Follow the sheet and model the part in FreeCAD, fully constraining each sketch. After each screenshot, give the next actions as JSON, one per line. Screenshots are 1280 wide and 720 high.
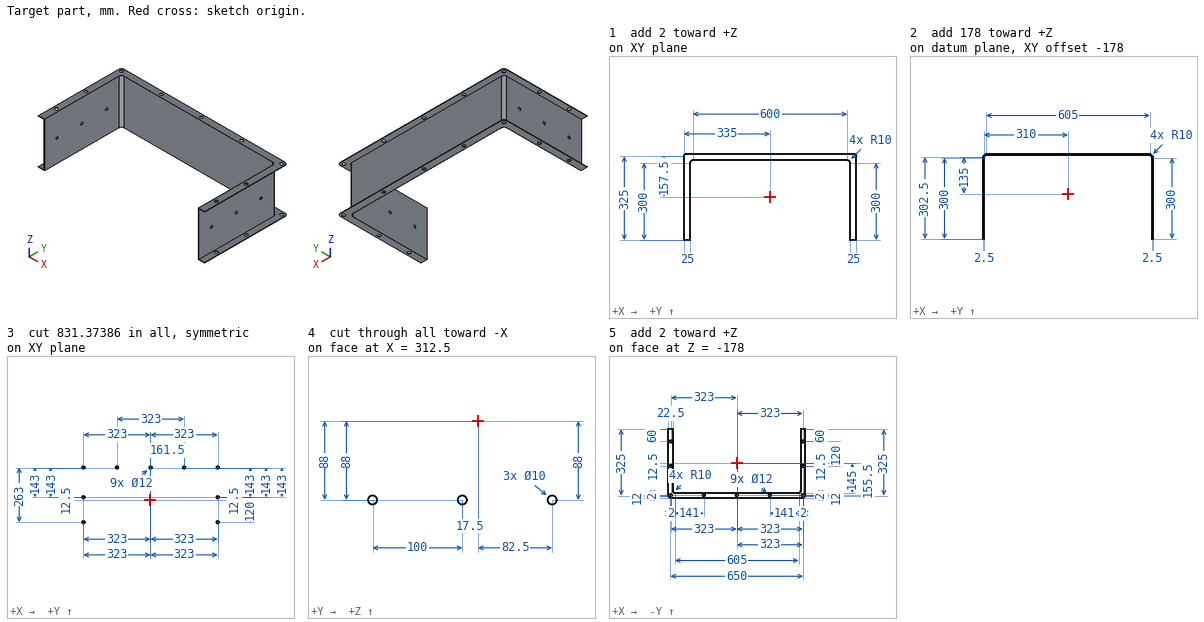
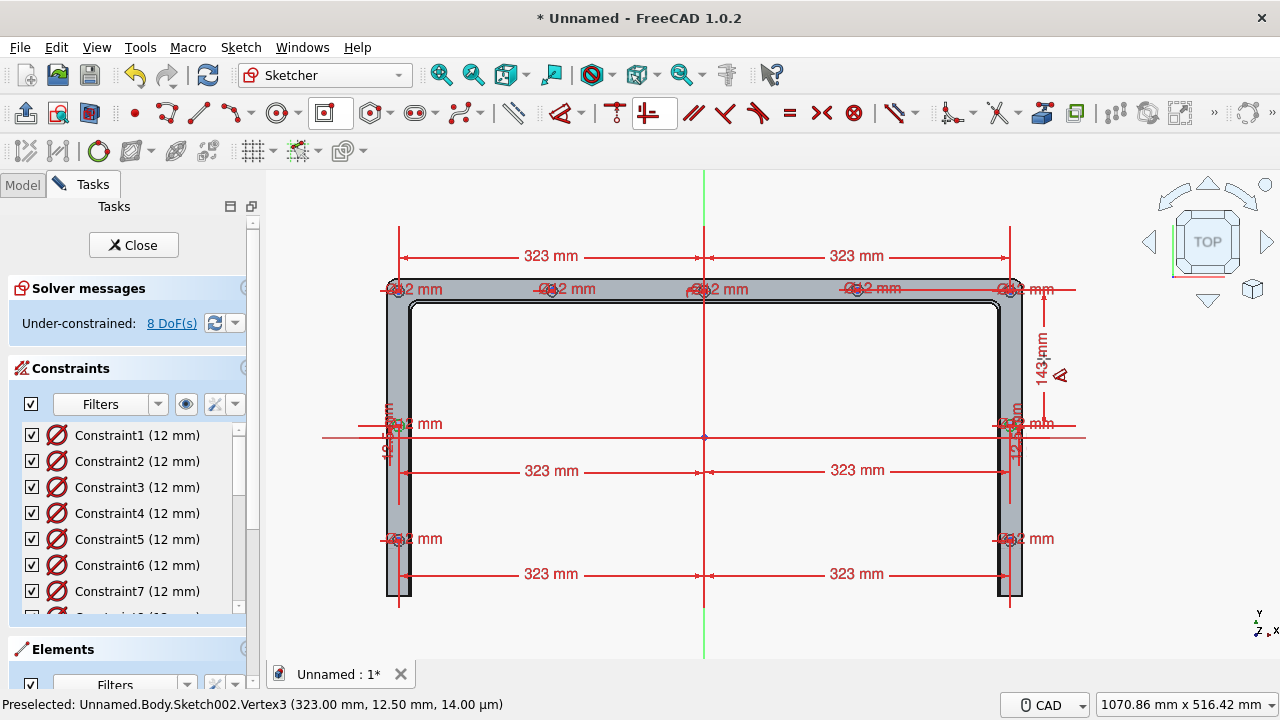
{"action": "left_click", "coordinate": [704, 291]}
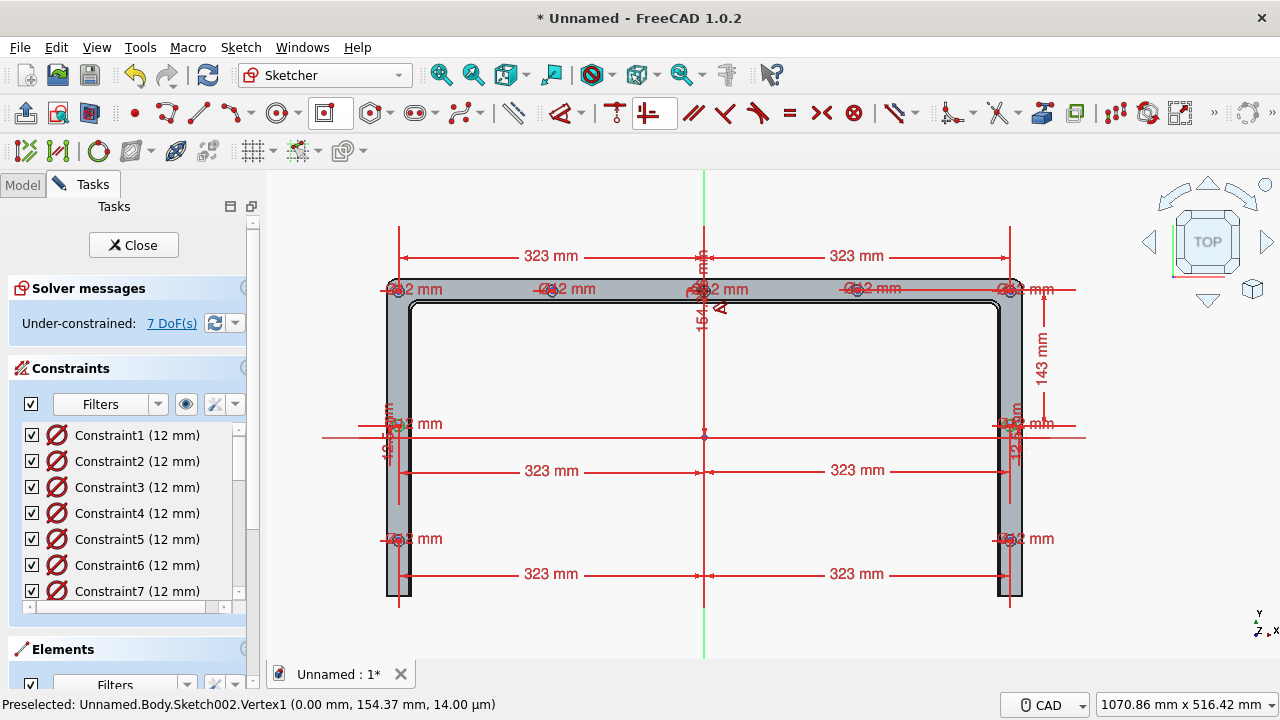
{"action": "left_click", "coordinate": [1010, 426]}
{"action": "left_click", "coordinate": [1044, 328]}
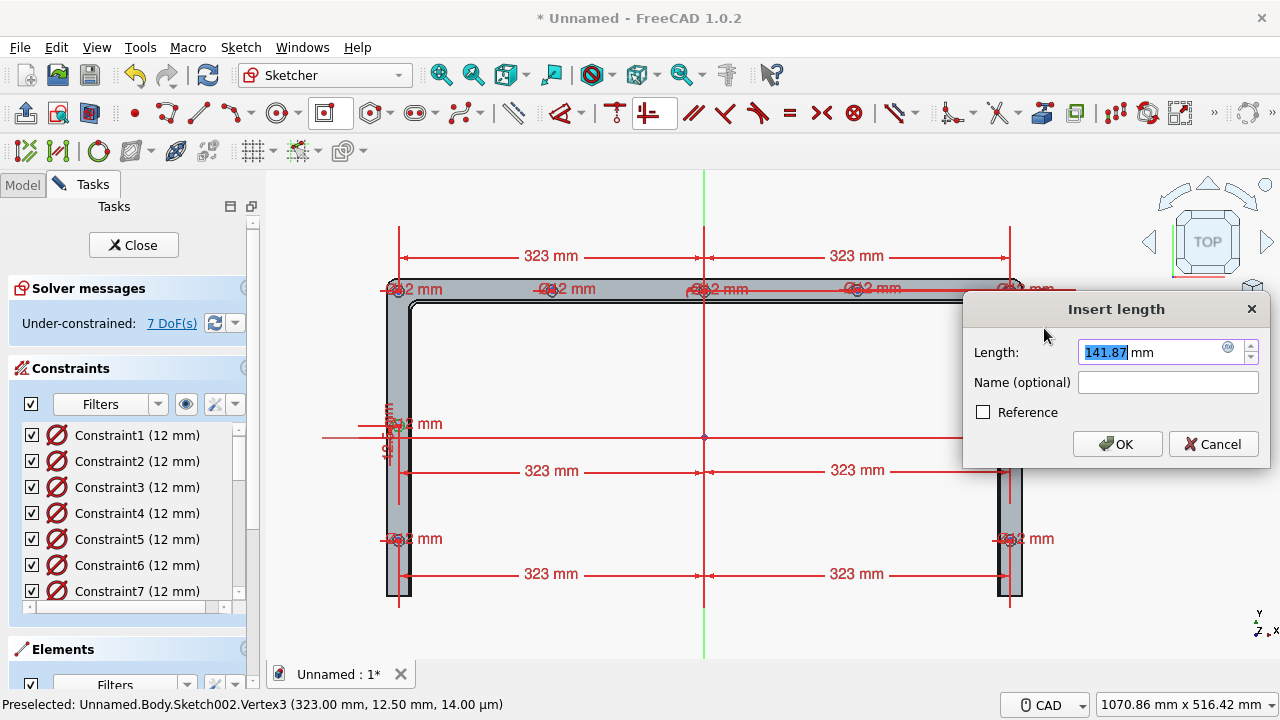
{"action": "type", "text": "143"}
{"action": "key", "text": "Return"}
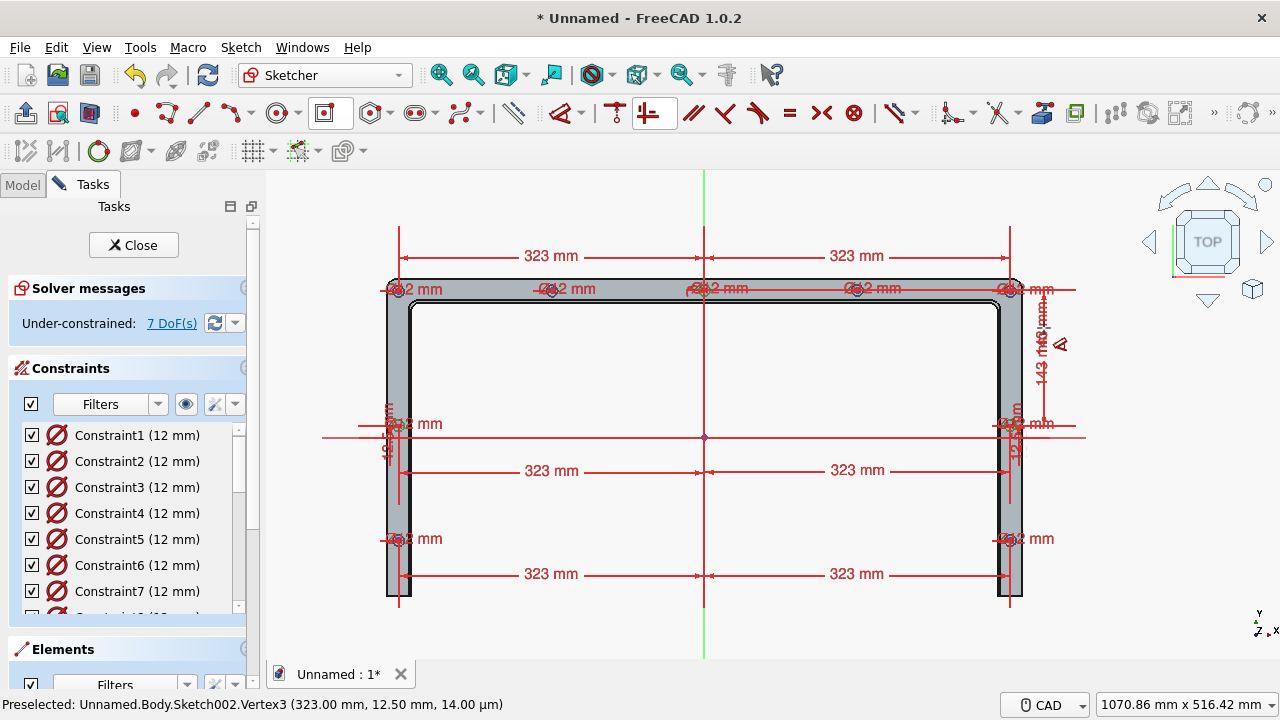
{"action": "left_click", "coordinate": [1010, 426]}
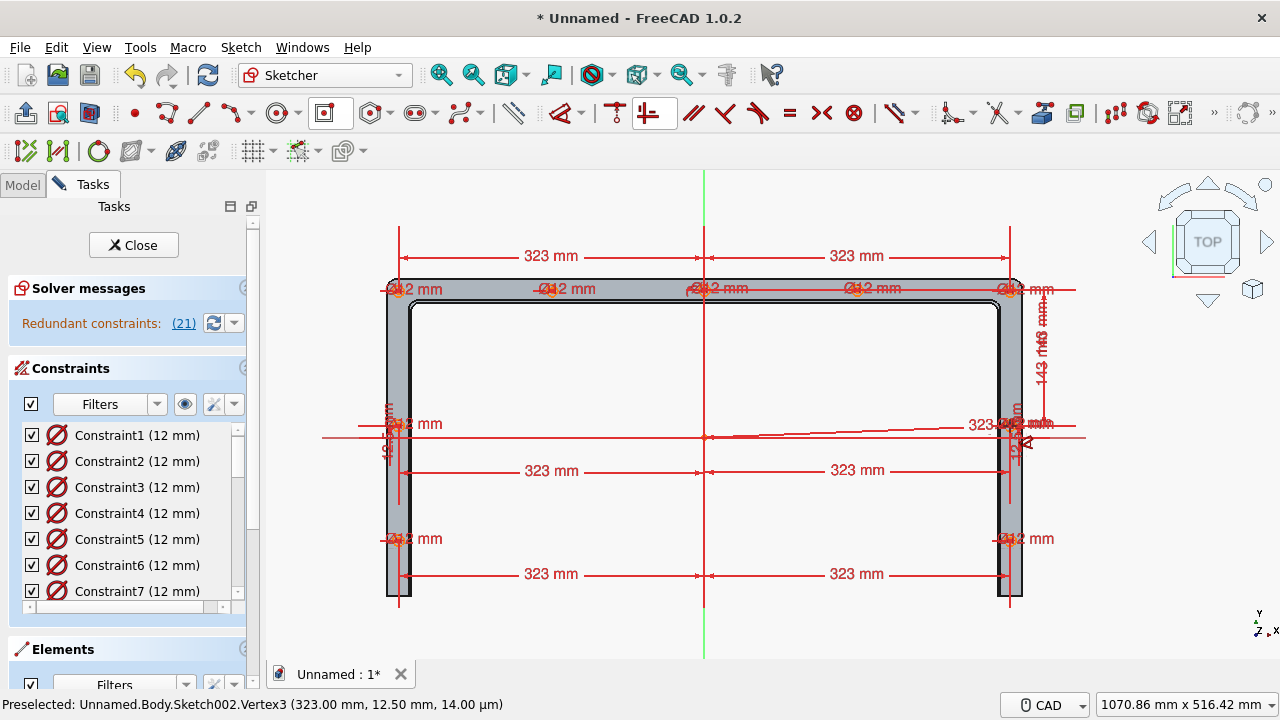
{"action": "left_click", "coordinate": [1010, 541]}
{"action": "left_click", "coordinate": [1044, 483]}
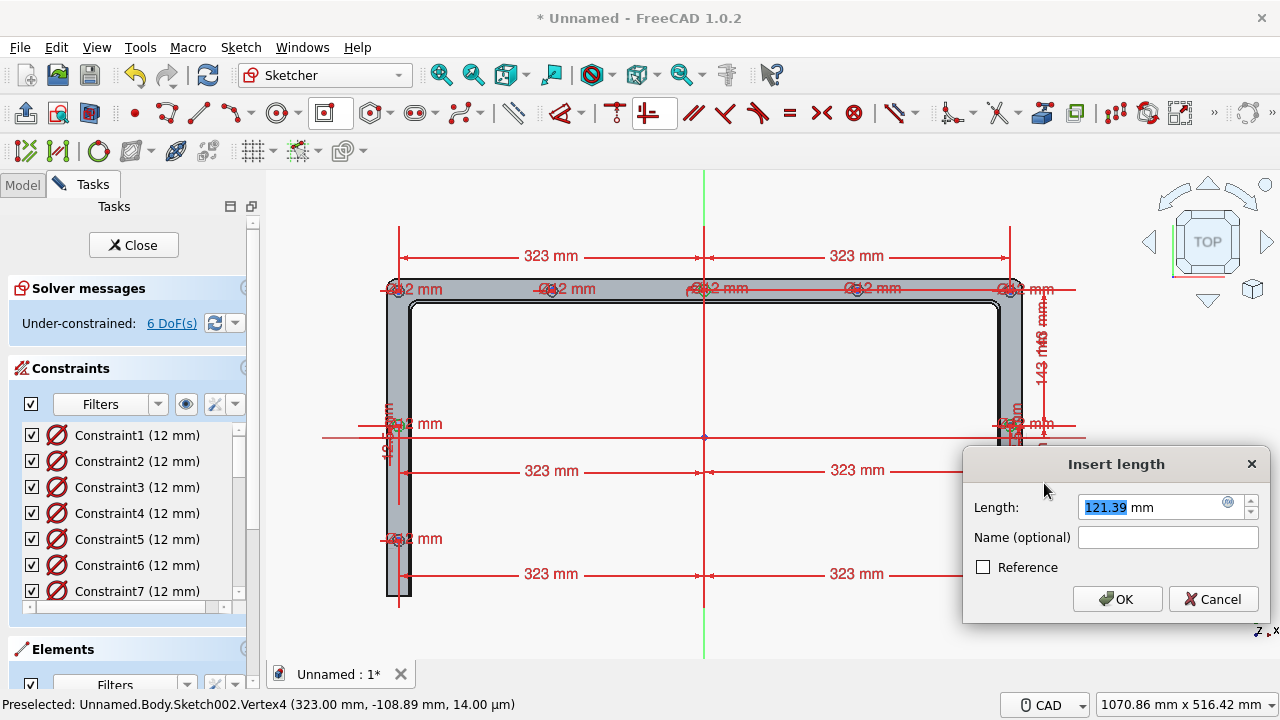
{"action": "type", "text": "120"}
{"action": "key", "text": "Return"}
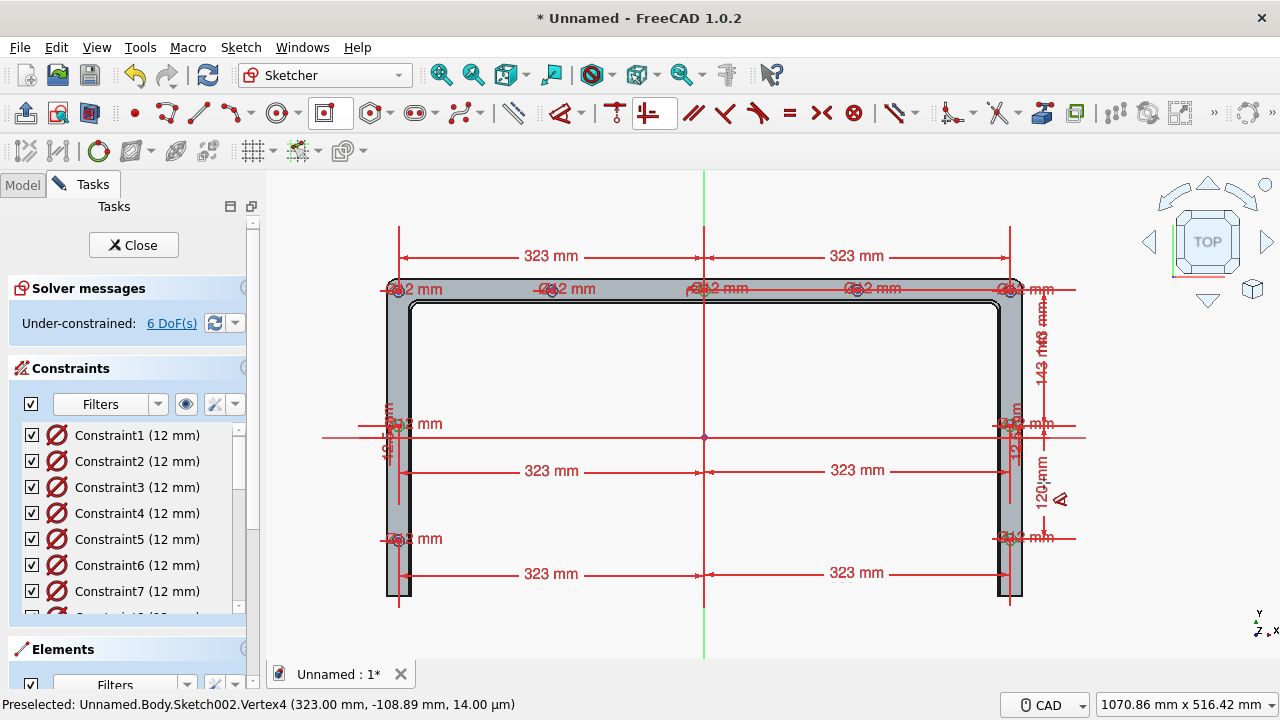
{"action": "left_click", "coordinate": [1010, 426]}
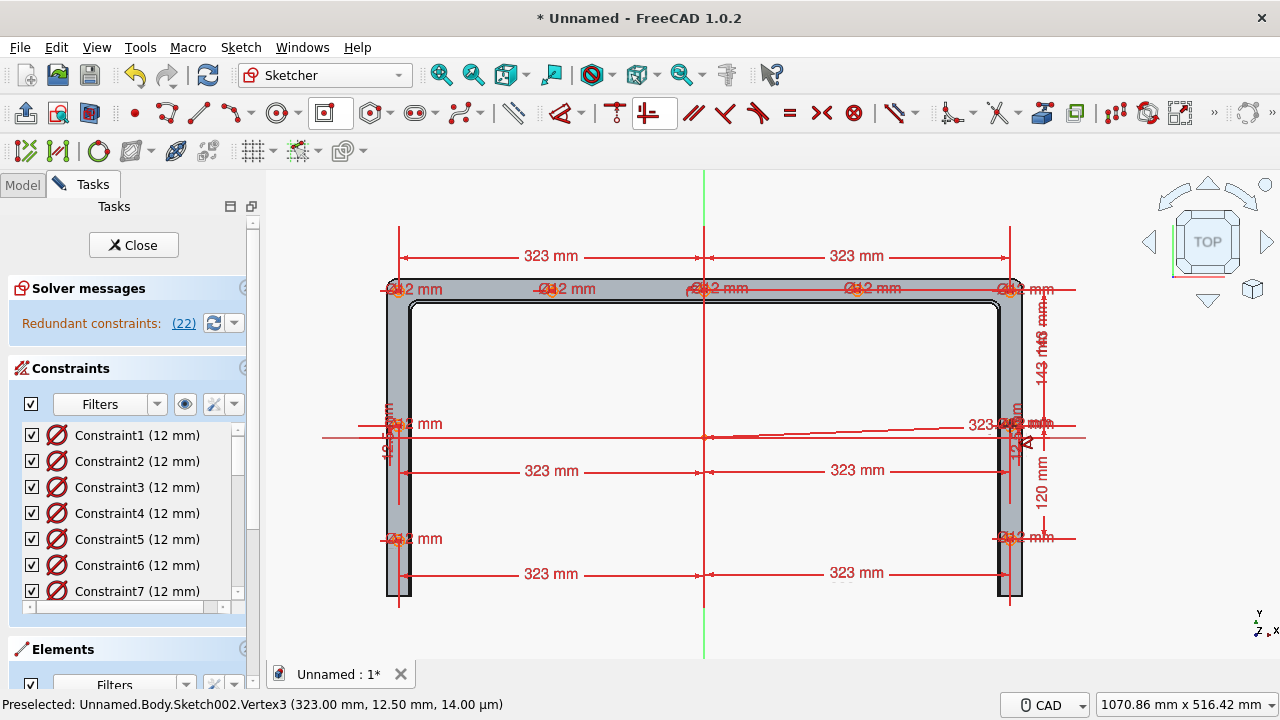
{"action": "left_click", "coordinate": [1010, 291]}
{"action": "left_click", "coordinate": [1044, 389]}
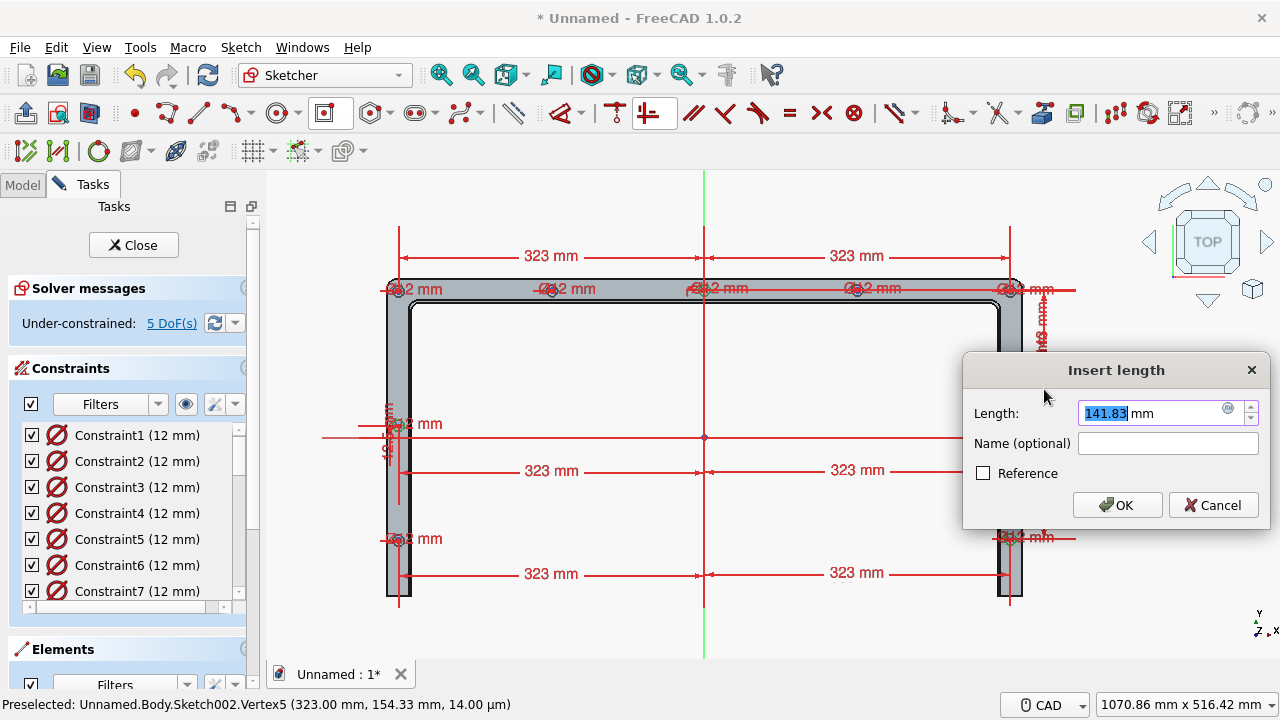
{"action": "type", "text": "143"}
{"action": "key", "text": "Return"}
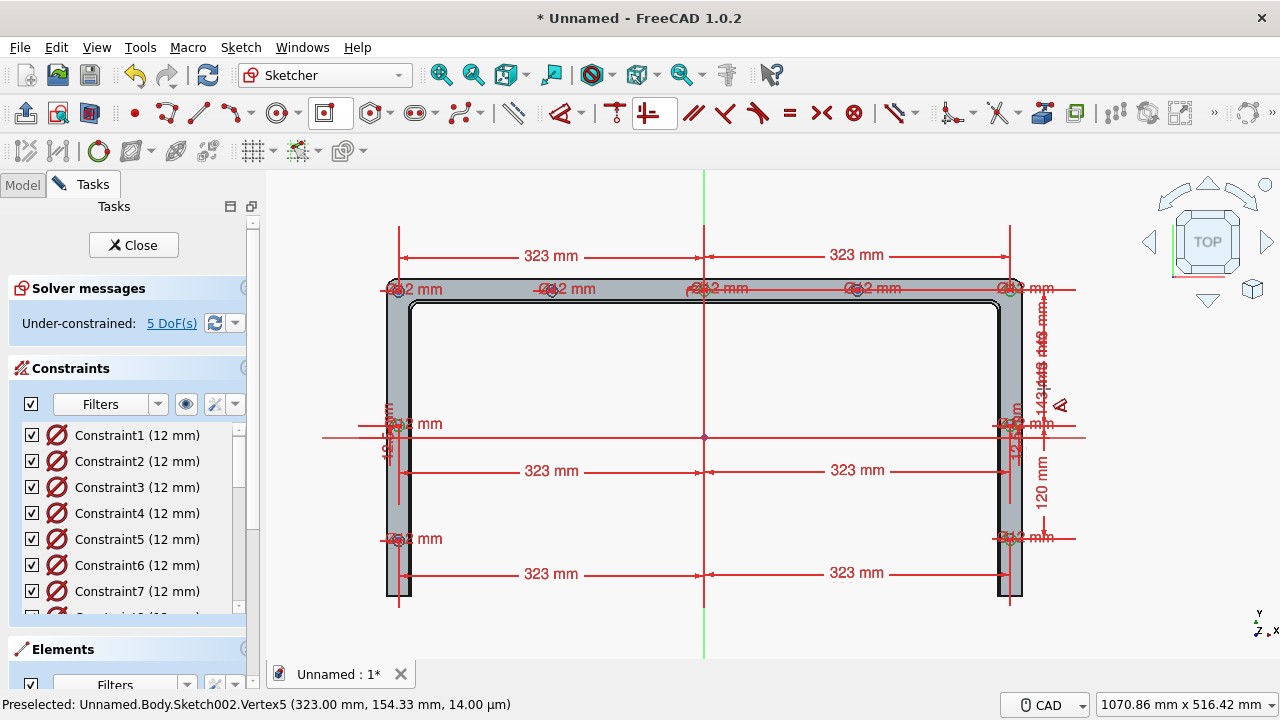
{"action": "left_click", "coordinate": [1010, 426]}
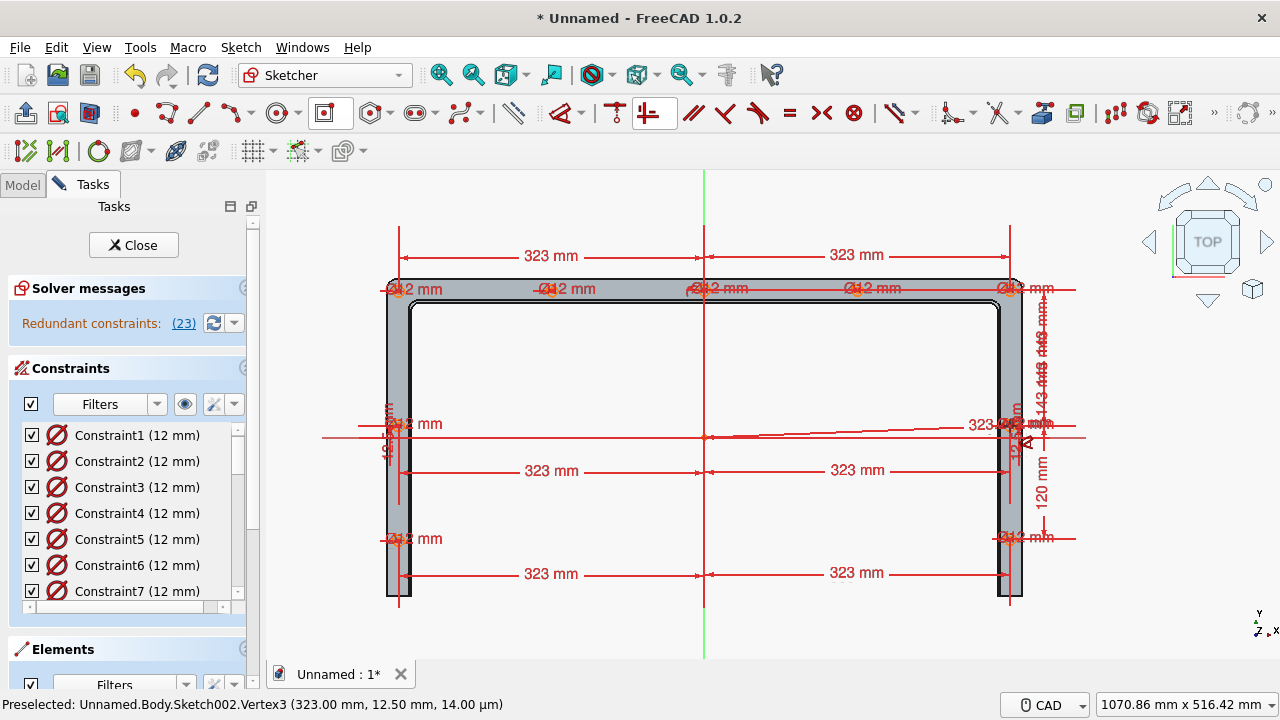
{"action": "left_click", "coordinate": [399, 291]}
{"action": "left_click", "coordinate": [365, 359]}